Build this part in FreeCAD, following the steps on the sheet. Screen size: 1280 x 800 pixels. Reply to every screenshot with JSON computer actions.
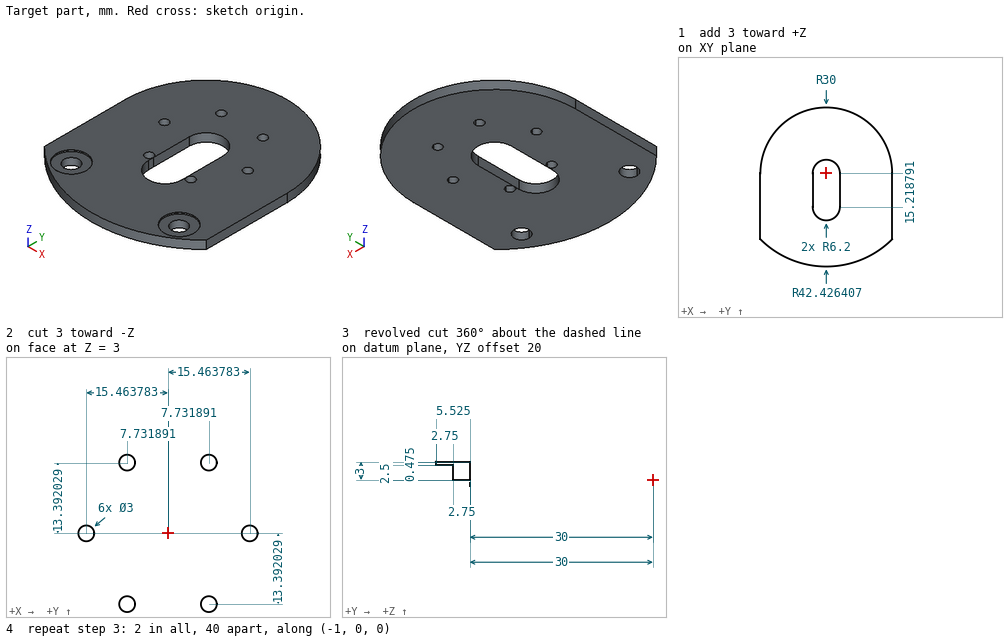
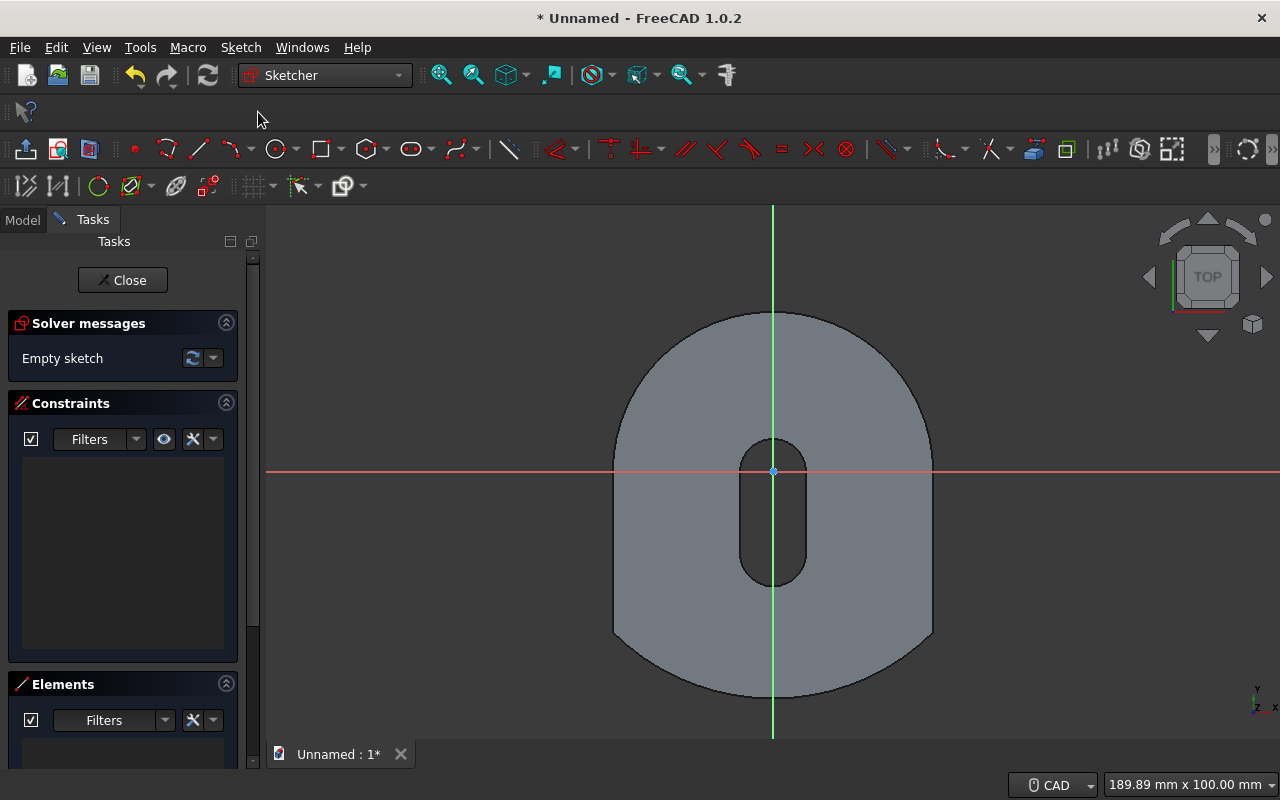
{"action": "scroll", "coordinate": [829, 472], "scroll_direction": "up", "scroll_amount": 4}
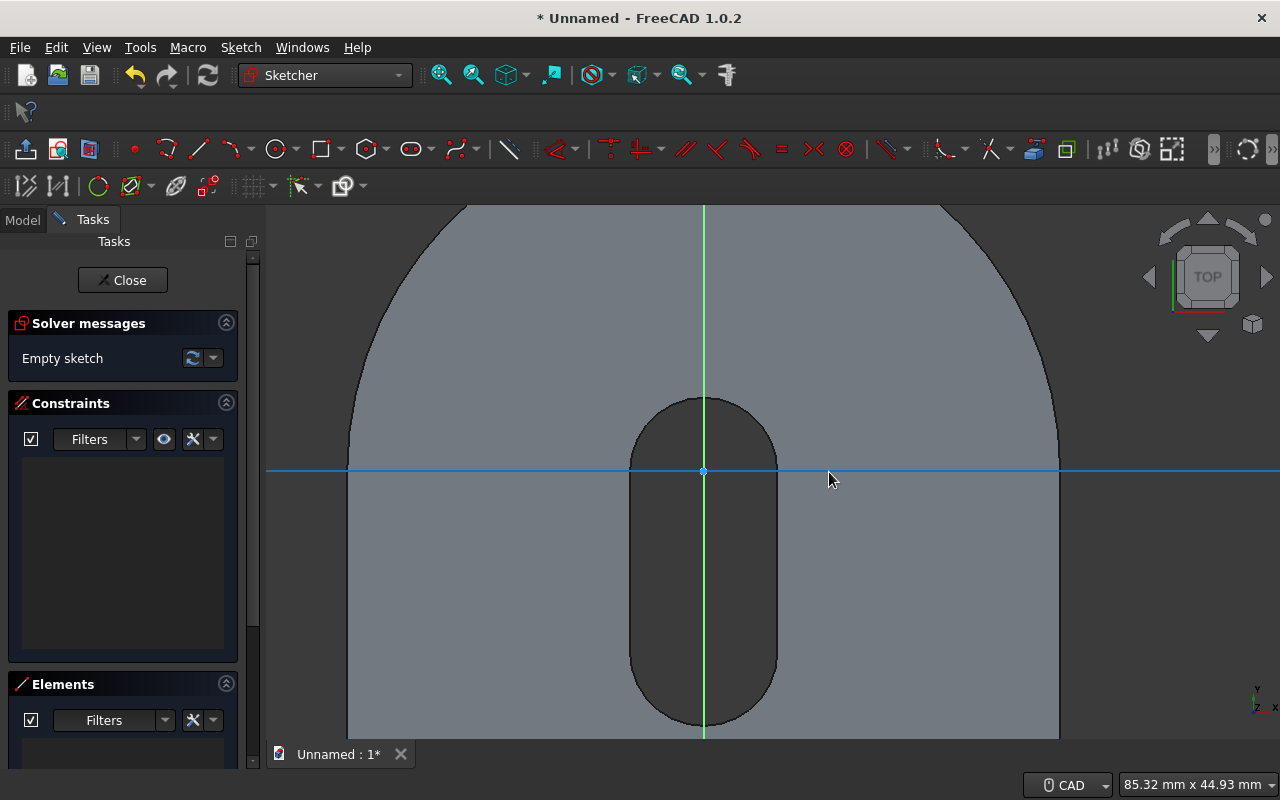
{"action": "key", "text": "g c"}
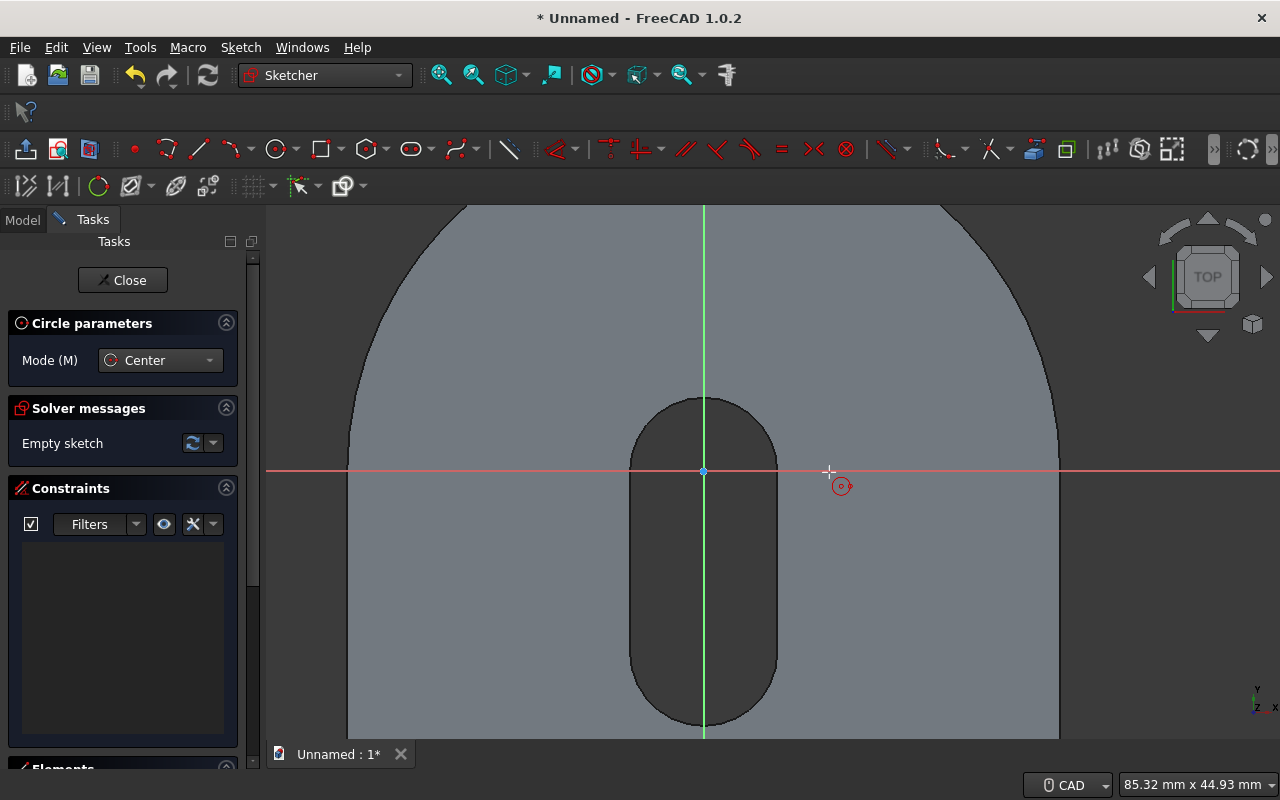
{"action": "scroll", "coordinate": [520, 471], "scroll_direction": "up", "scroll_amount": 2}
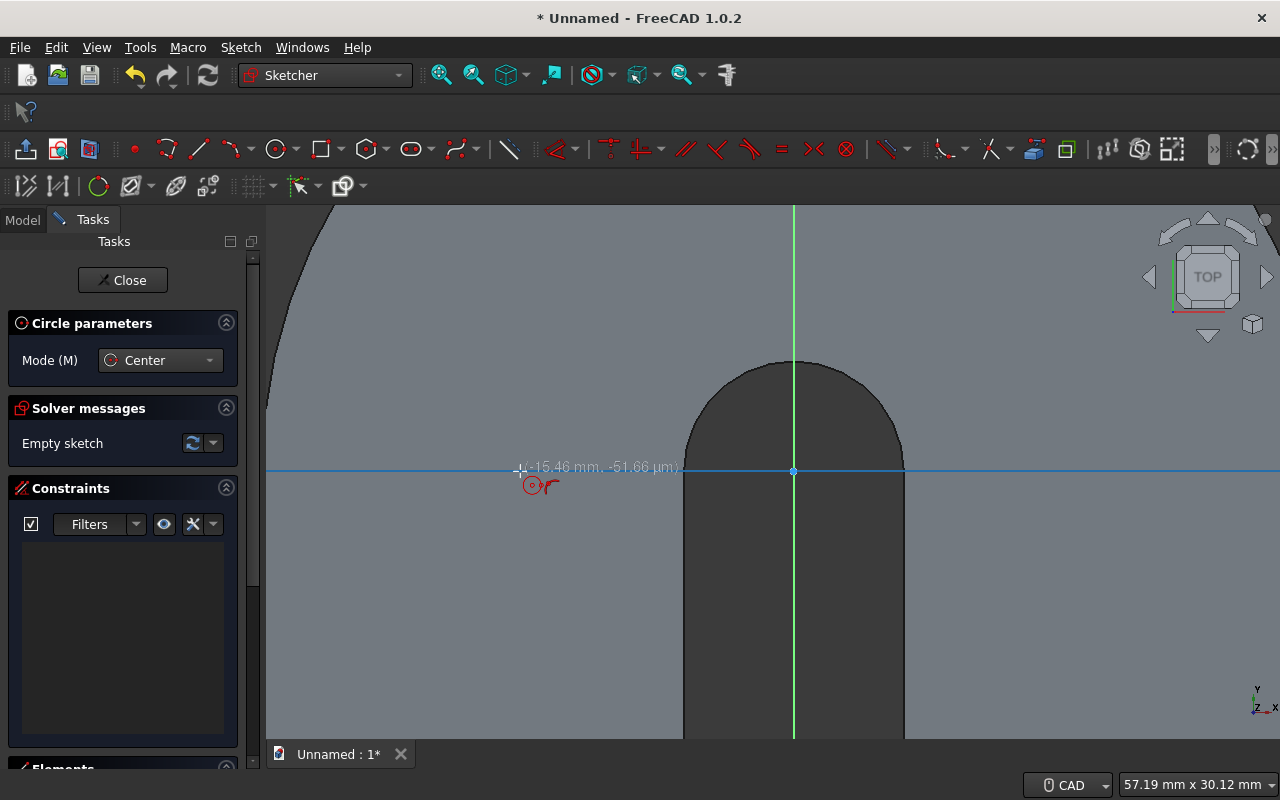
{"action": "left_click", "coordinate": [520, 471]}
{"action": "mouse_move", "coordinate": [539, 453]}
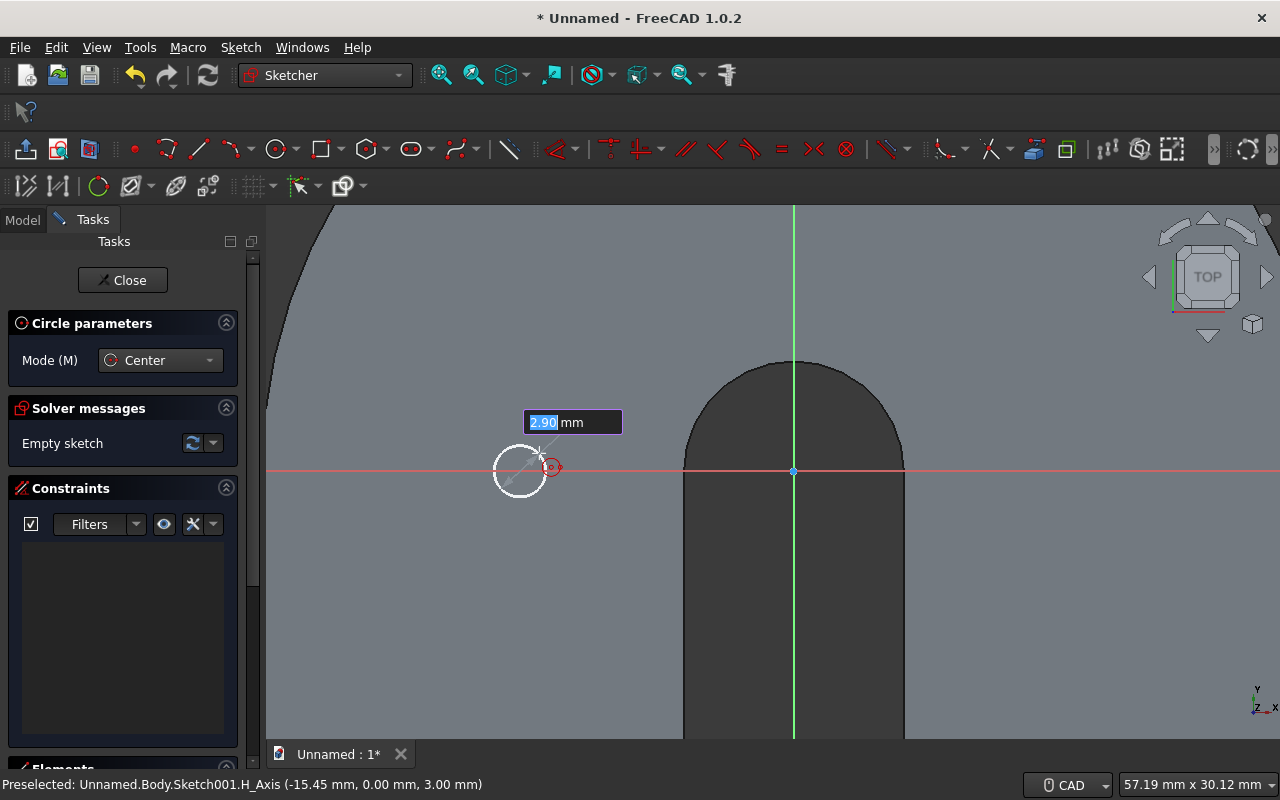
{"action": "type", "text": "3"}
{"action": "key", "text": "Return"}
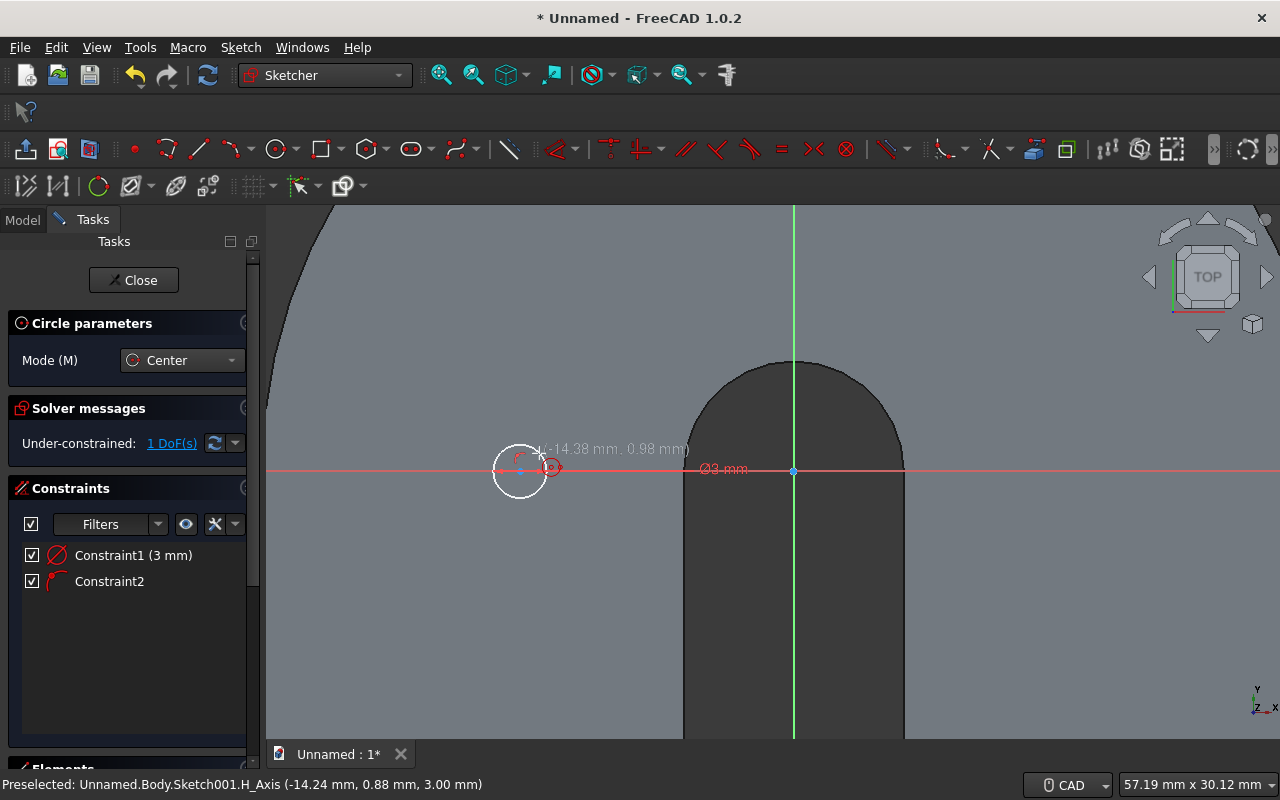
{"action": "left_click", "coordinate": [657, 234]}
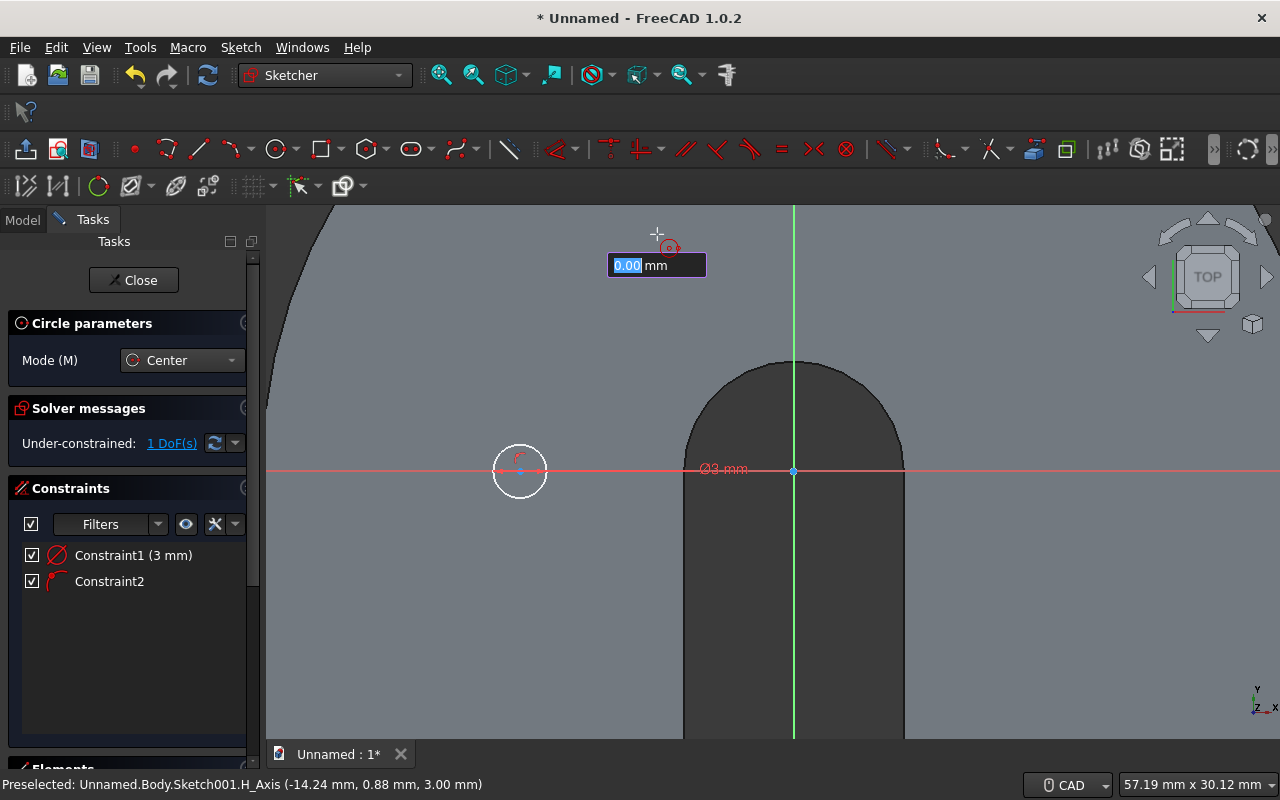
{"action": "scroll", "coordinate": [523, 473], "scroll_direction": "down", "scroll_amount": 2}
{"action": "mouse_move", "coordinate": [625, 300]}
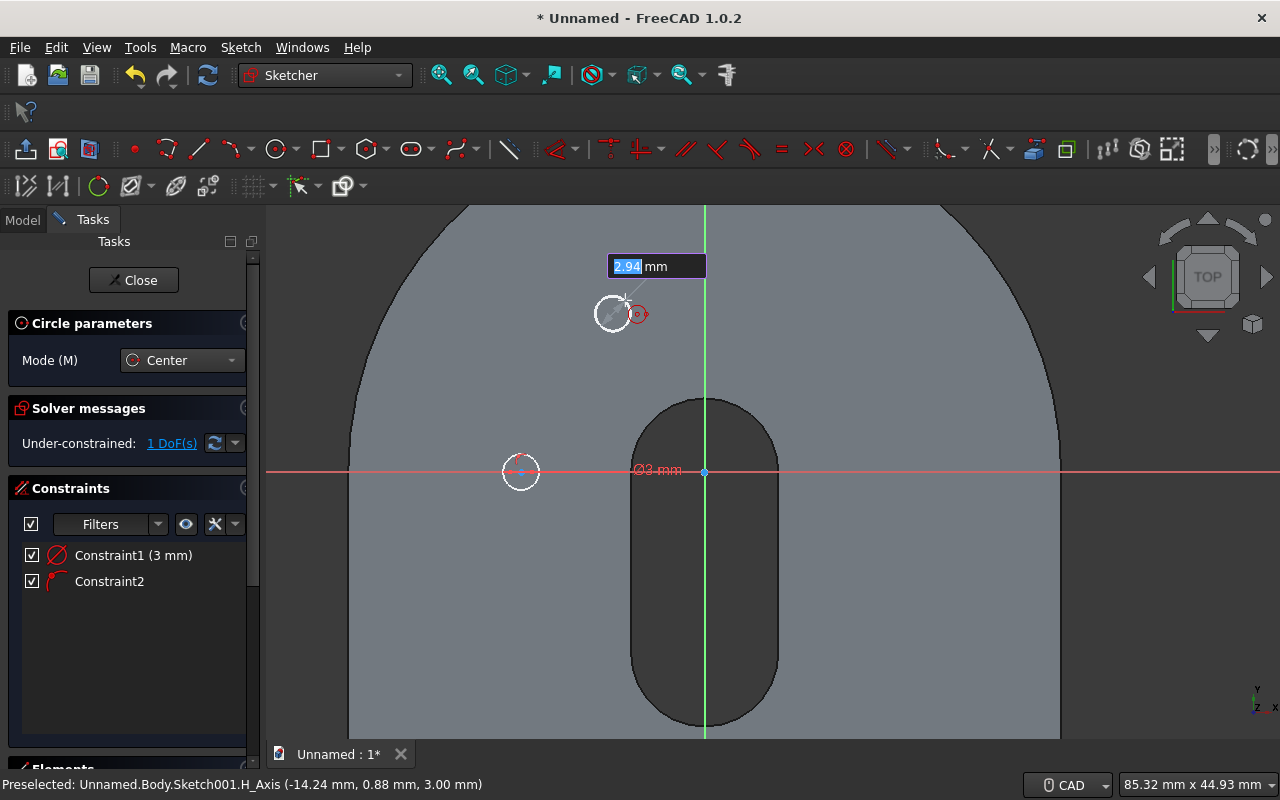
{"action": "type", "text": "3"}
{"action": "key", "text": "Return"}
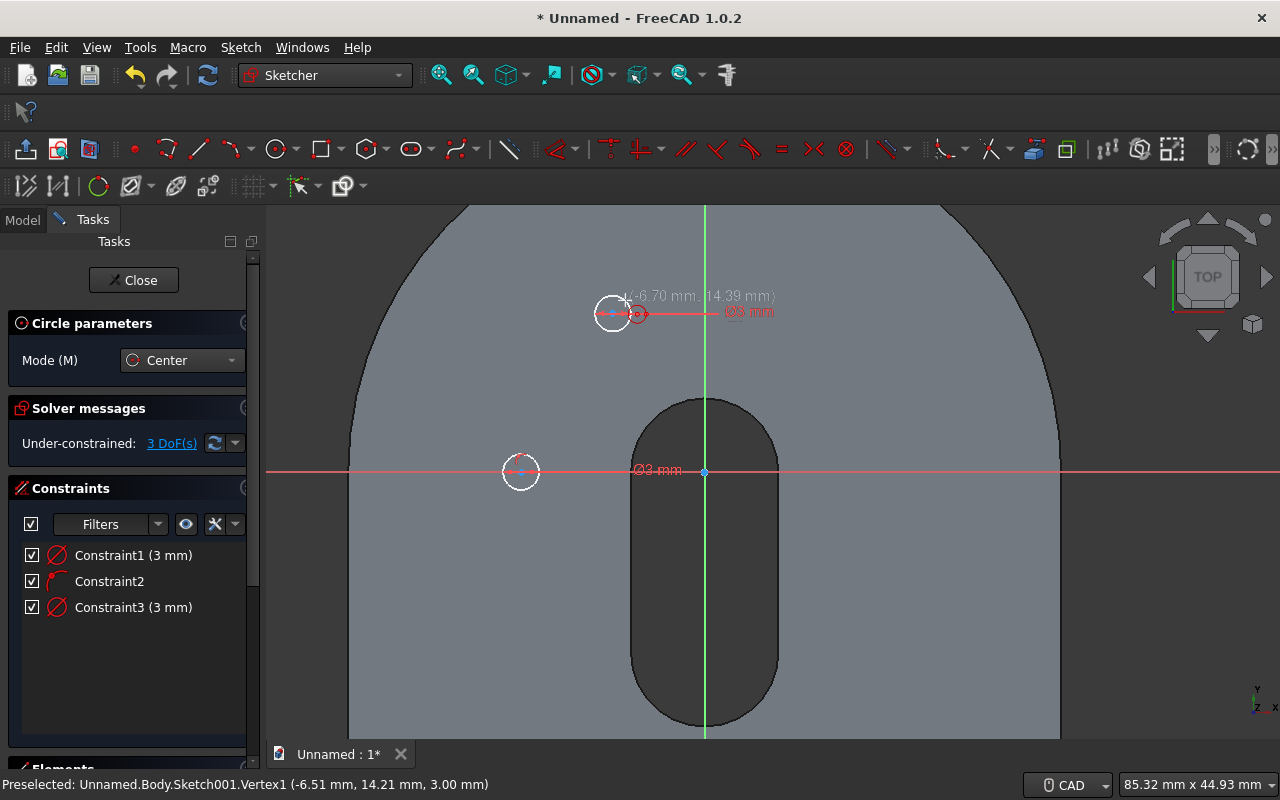
{"action": "scroll", "coordinate": [797, 313], "scroll_direction": "up", "scroll_amount": 2}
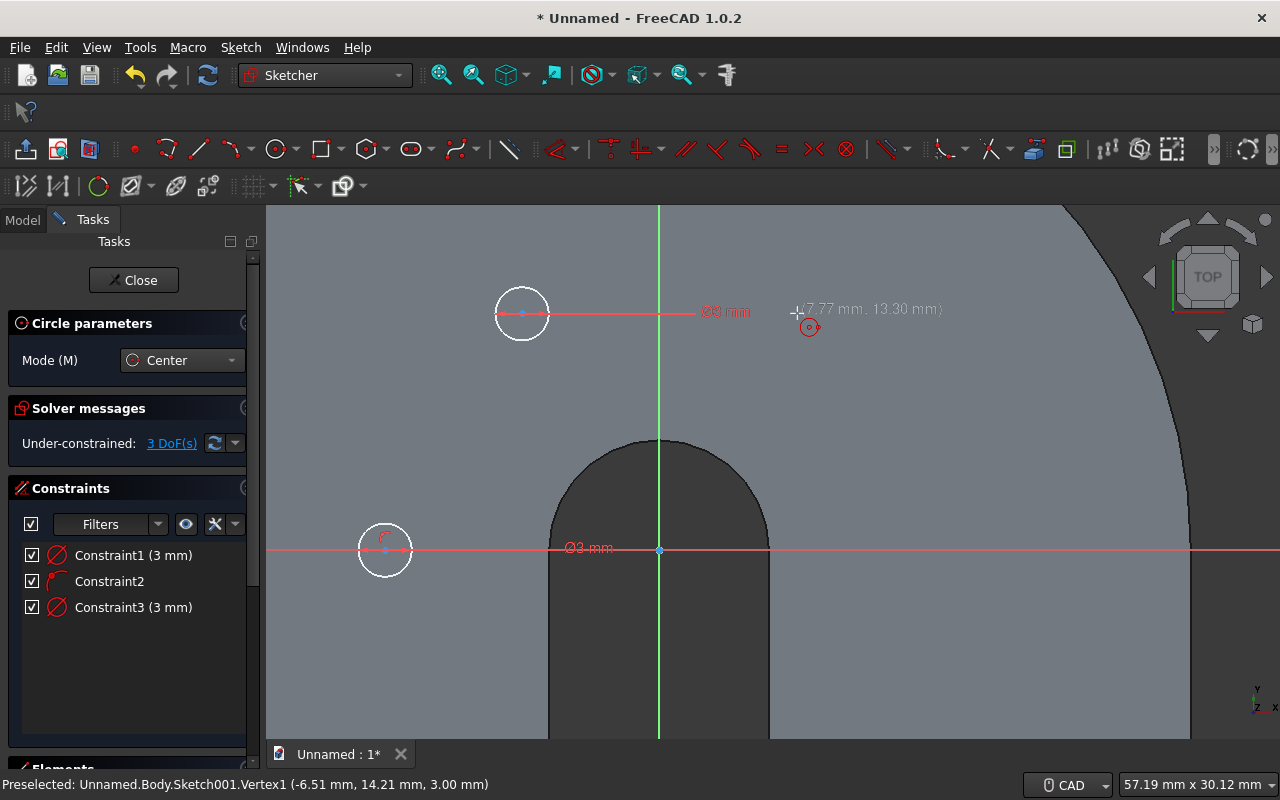
{"action": "left_click", "coordinate": [796, 313]}
{"action": "mouse_move", "coordinate": [815, 294]}